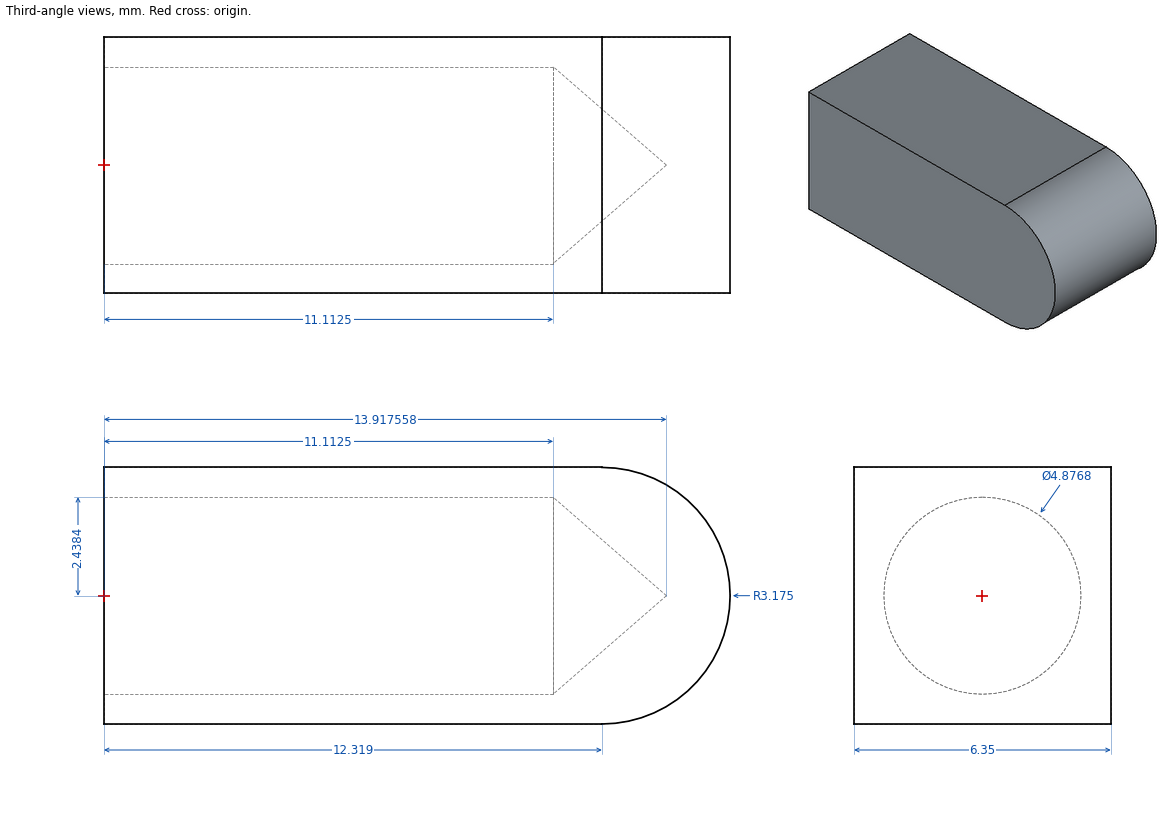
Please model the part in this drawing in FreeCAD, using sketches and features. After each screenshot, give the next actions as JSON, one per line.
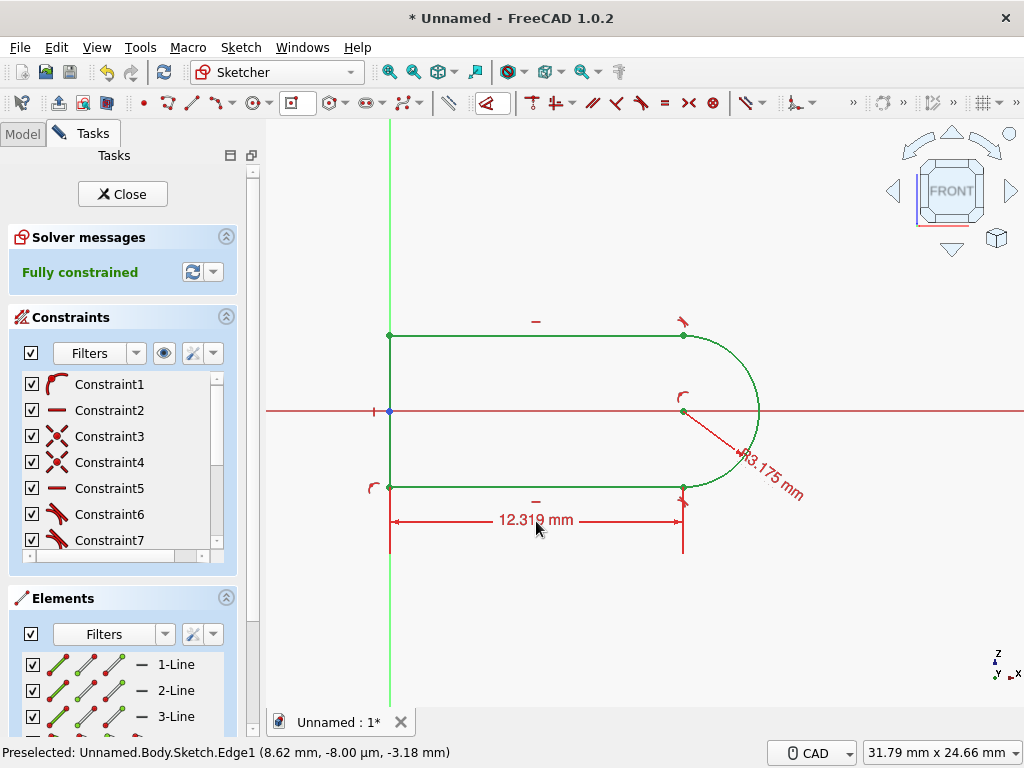
{"action": "left_click", "coordinate": [123, 194]}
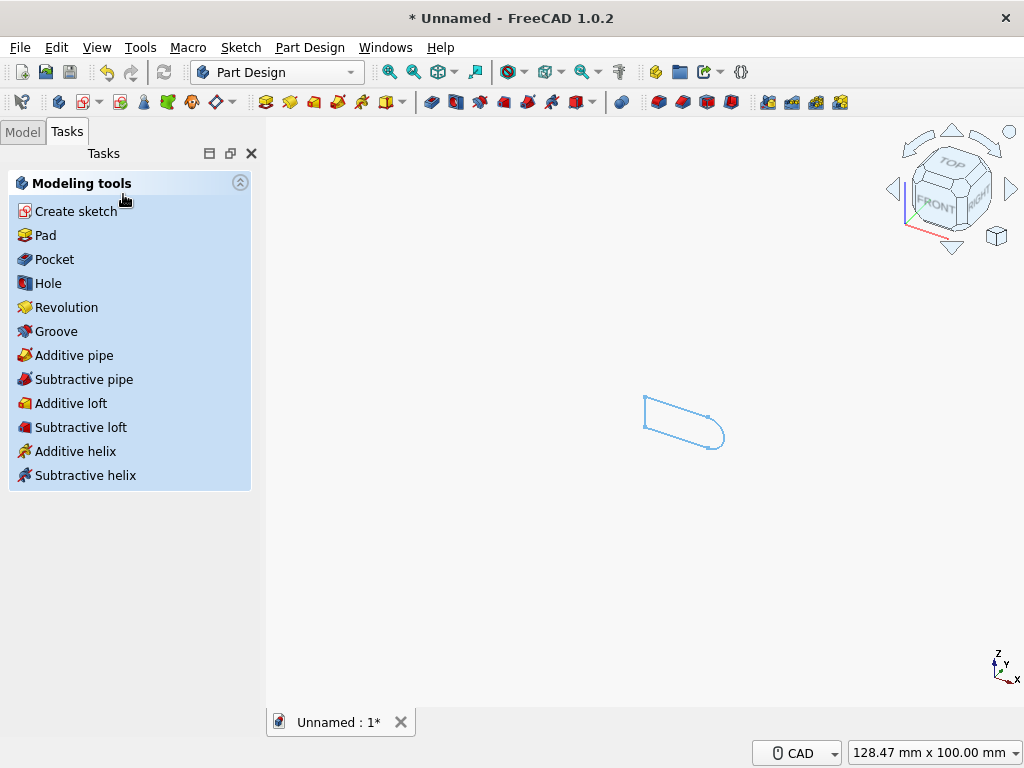
{"action": "left_click", "coordinate": [266, 102]}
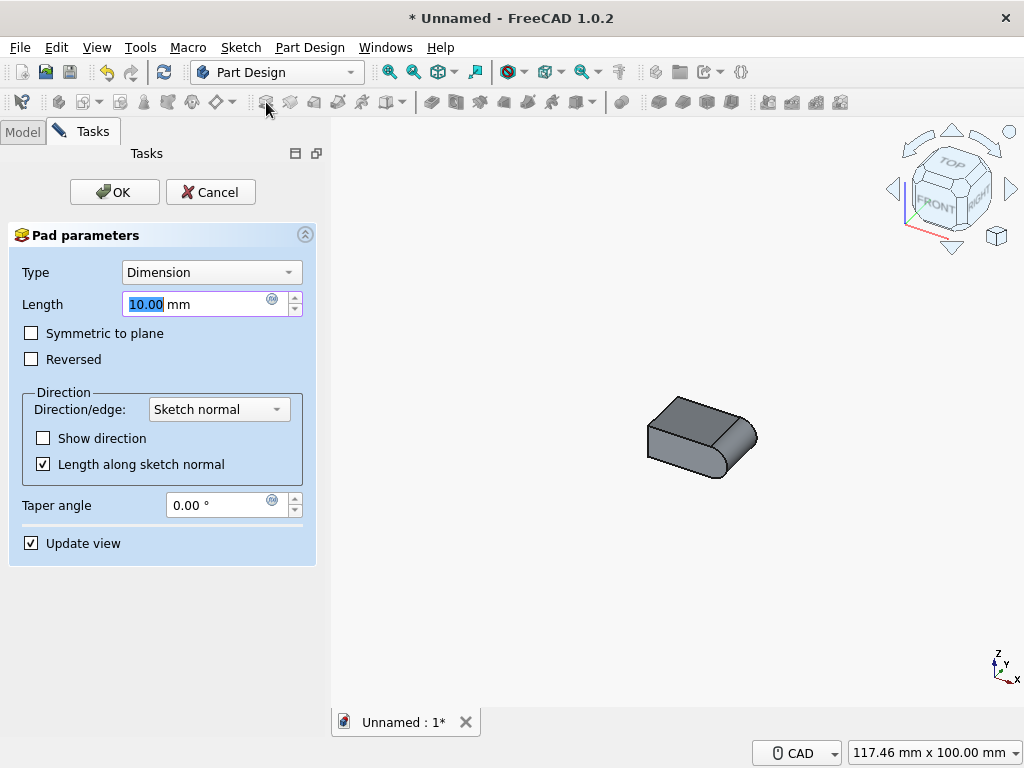
{"action": "type", "text": "6.35"}
{"action": "key", "text": "Tab"}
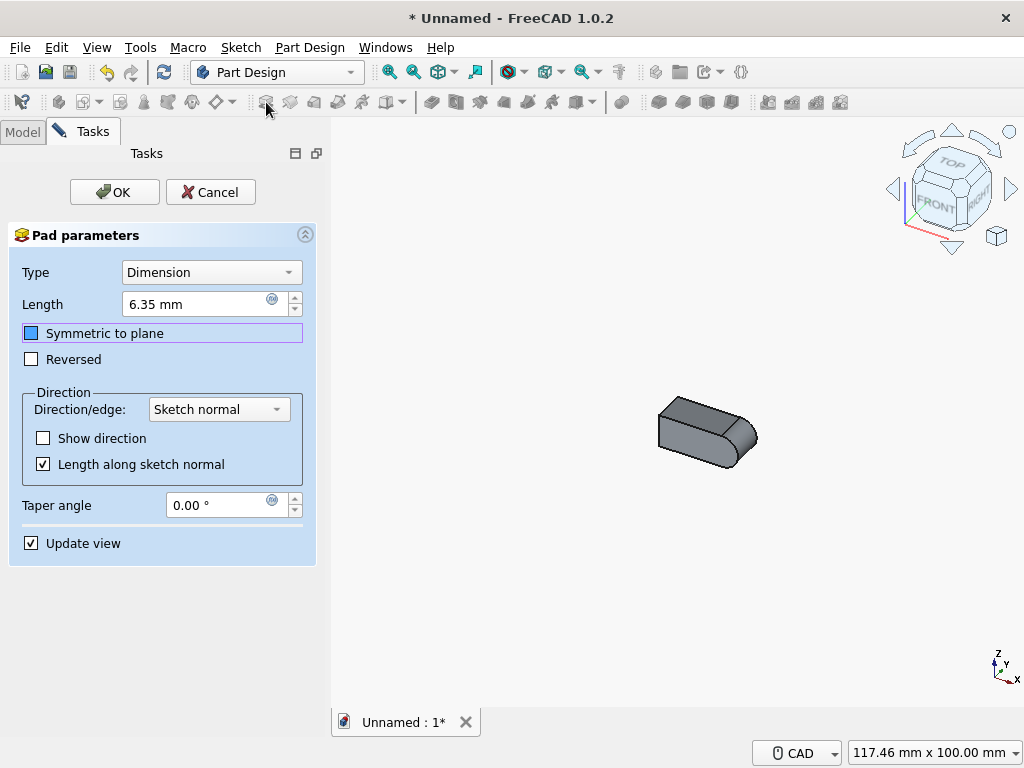
{"action": "left_click", "coordinate": [30, 333]}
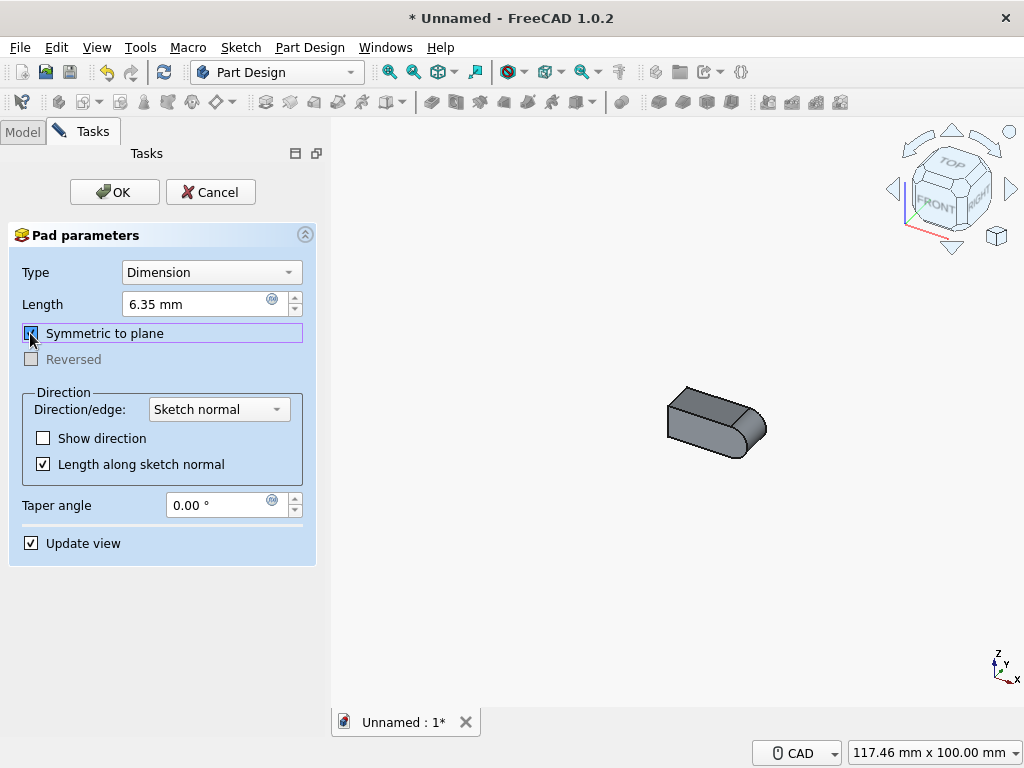
{"action": "left_click", "coordinate": [115, 192]}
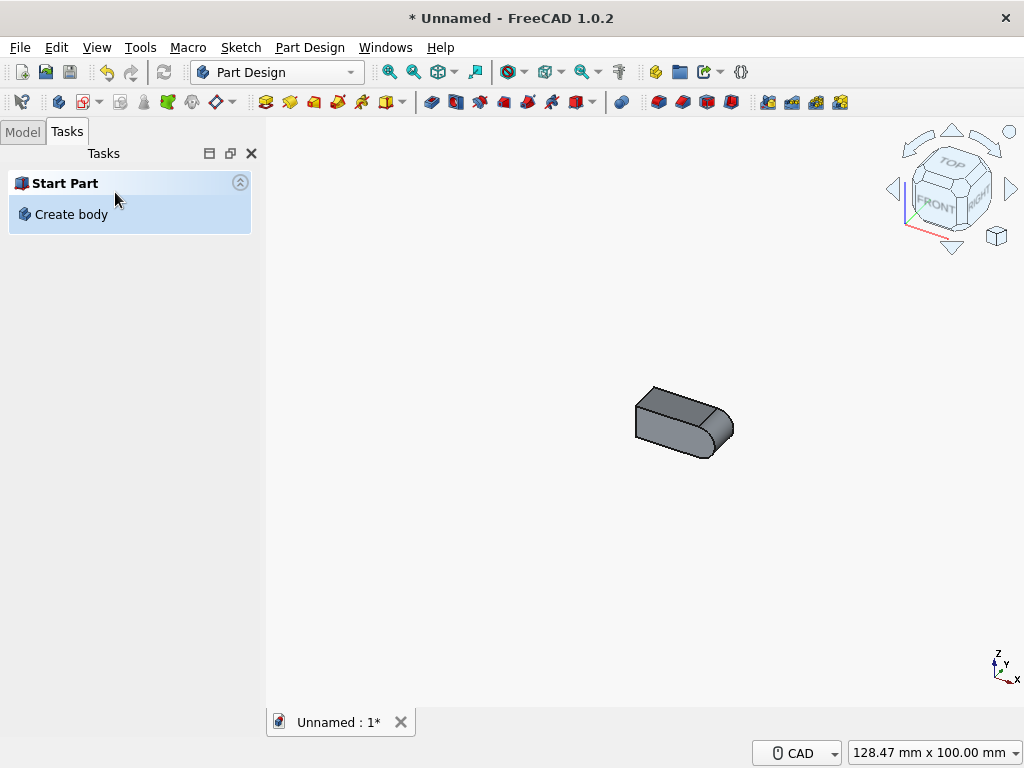
{"action": "key", "text": "v f"}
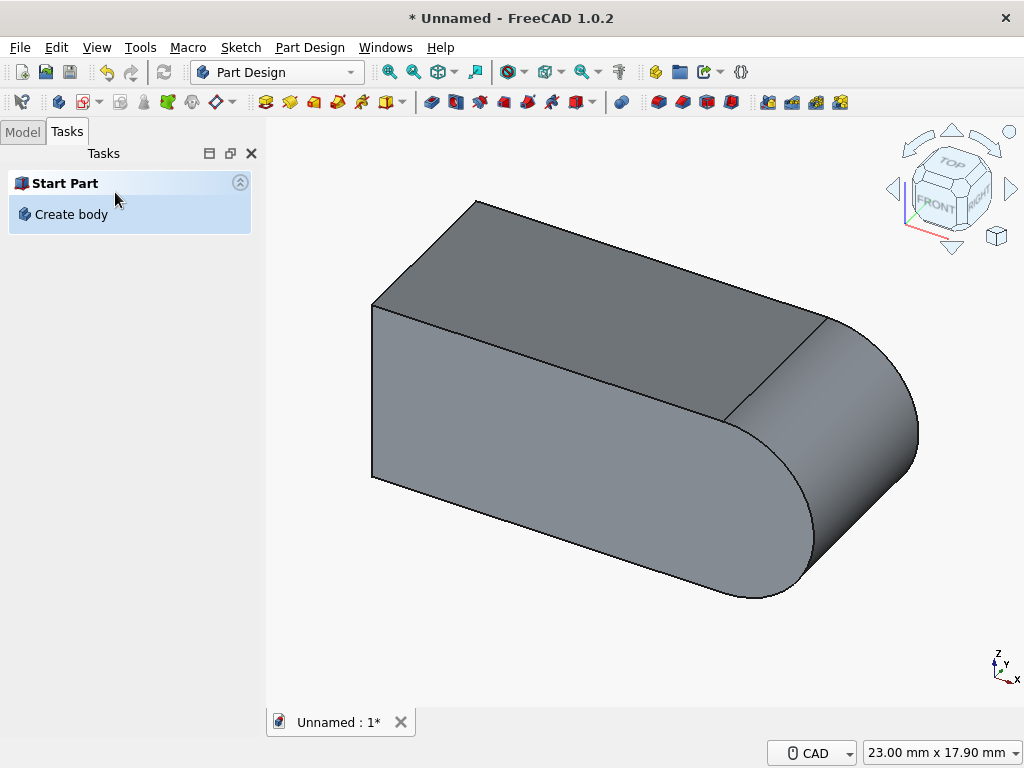
{"action": "key", "text": "6"}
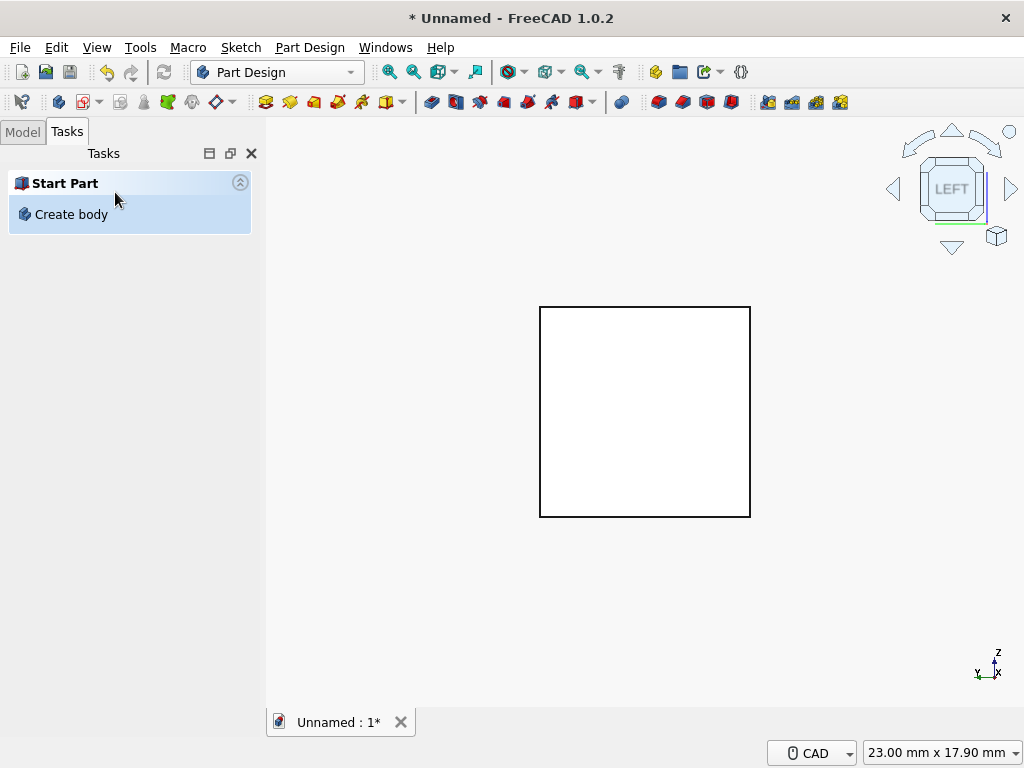
{"action": "left_click", "coordinate": [390, 72]}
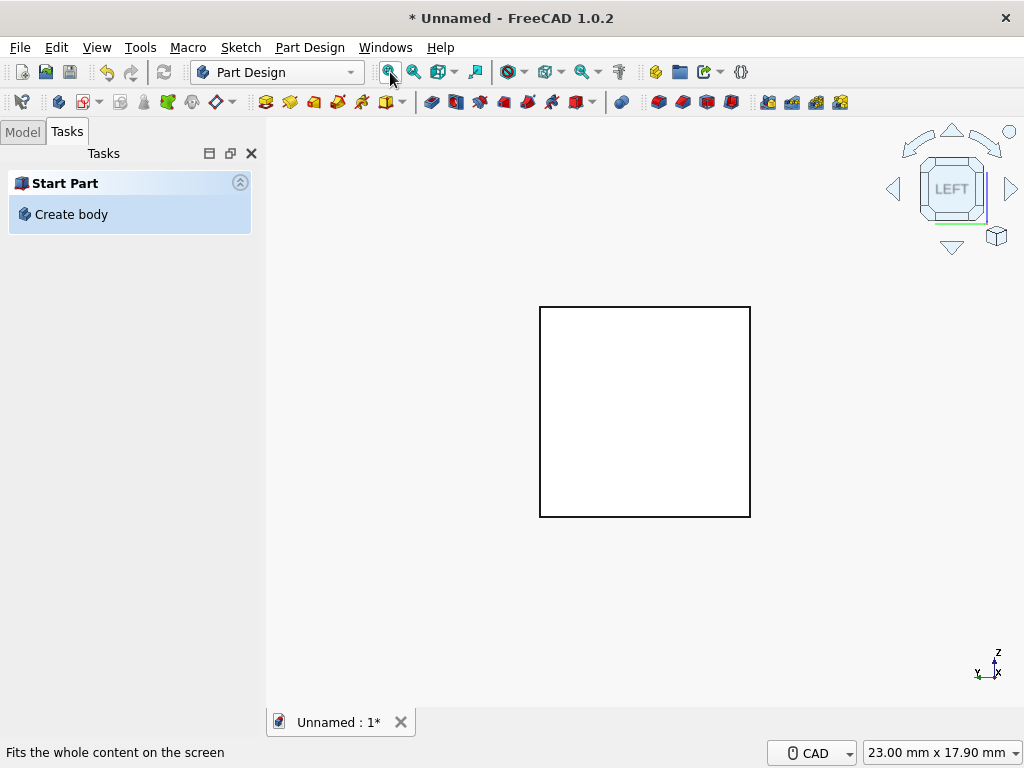
{"action": "left_click", "coordinate": [645, 411]}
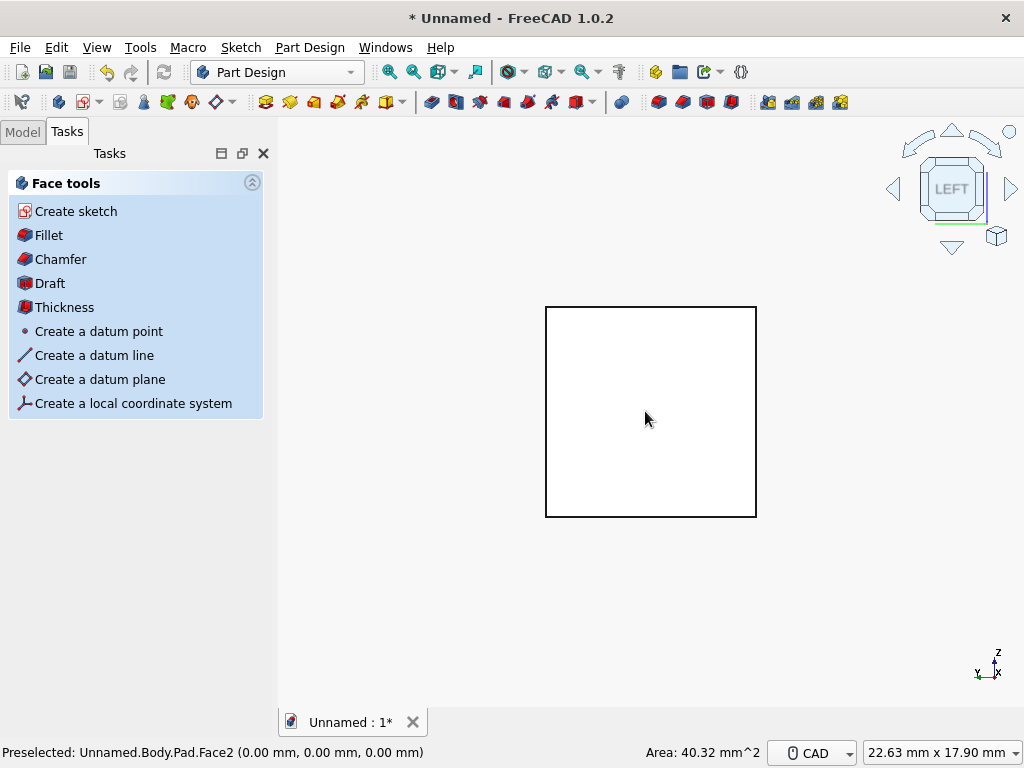
{"action": "left_click", "coordinate": [84, 102]}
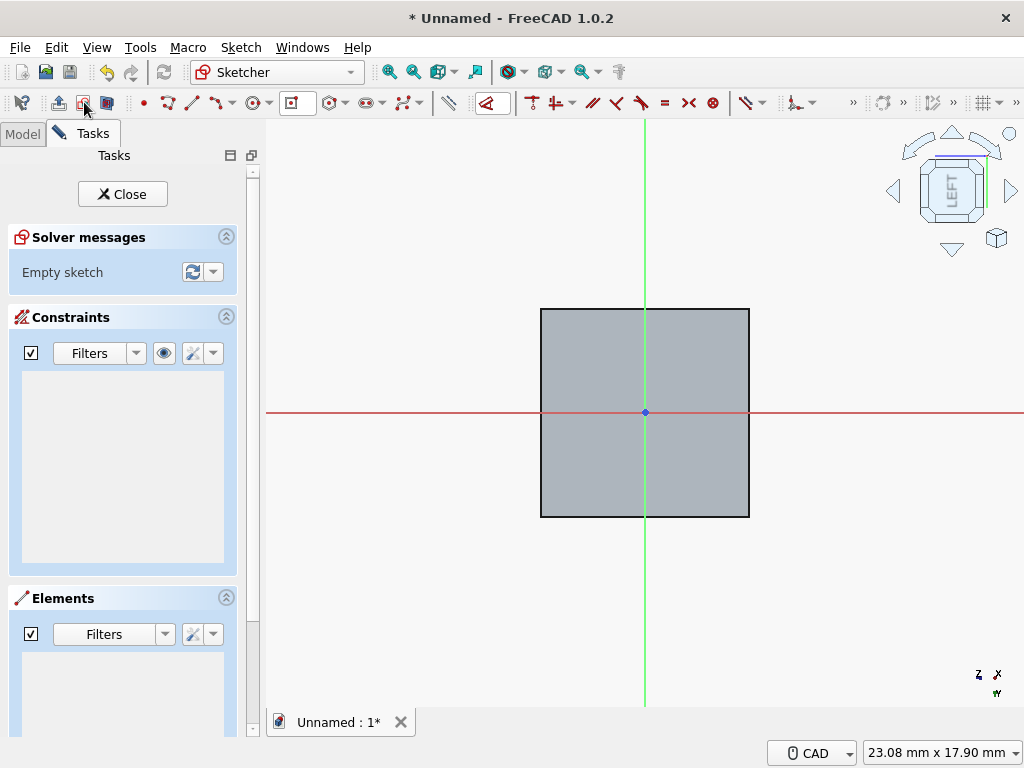
{"action": "scroll", "coordinate": [701, 413], "scroll_direction": "up", "scroll_amount": 4}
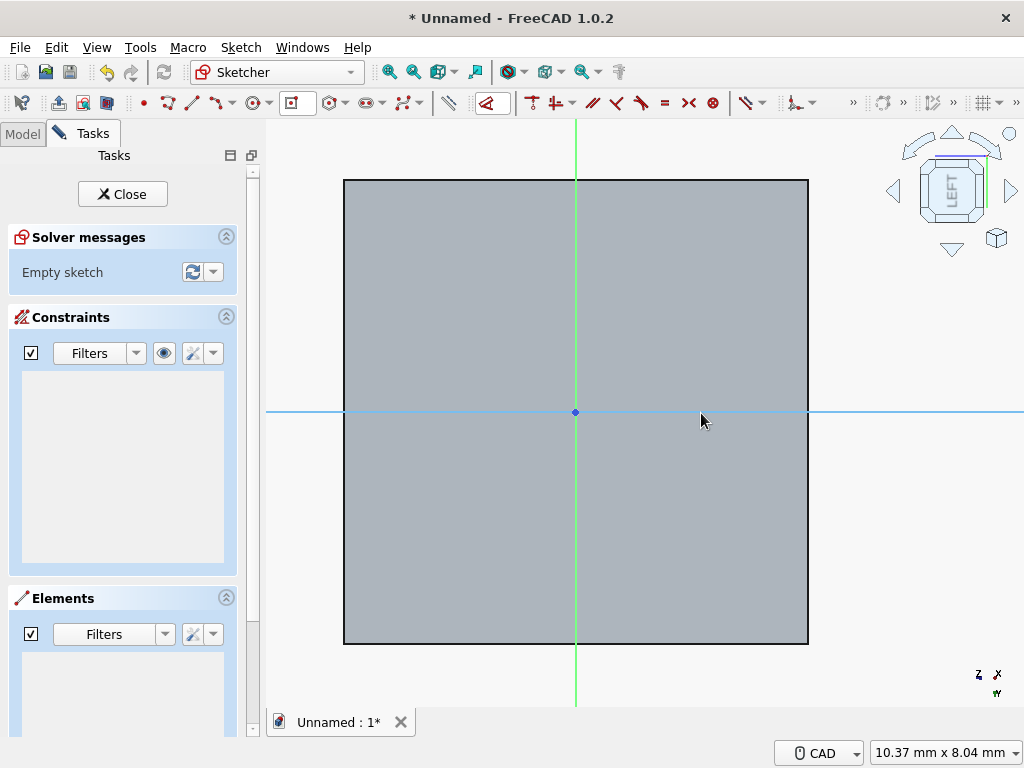
{"action": "key", "text": "g c"}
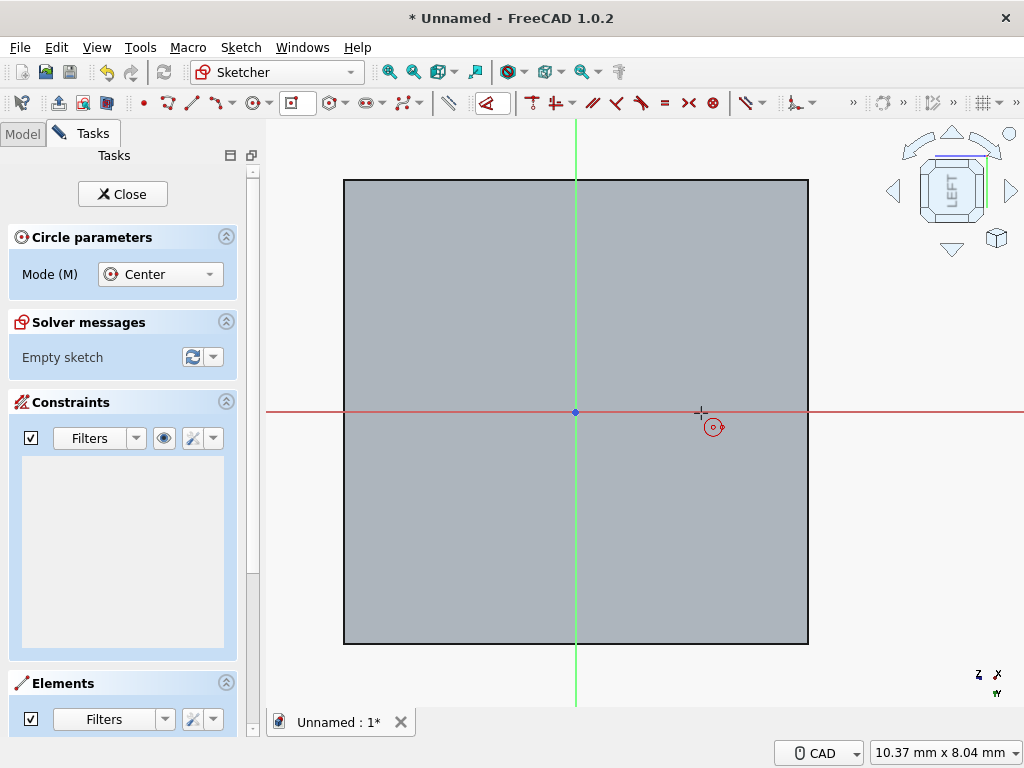
{"action": "left_click", "coordinate": [576, 412]}
{"action": "left_click", "coordinate": [702, 286]}
{"action": "key", "text": "Escape"}